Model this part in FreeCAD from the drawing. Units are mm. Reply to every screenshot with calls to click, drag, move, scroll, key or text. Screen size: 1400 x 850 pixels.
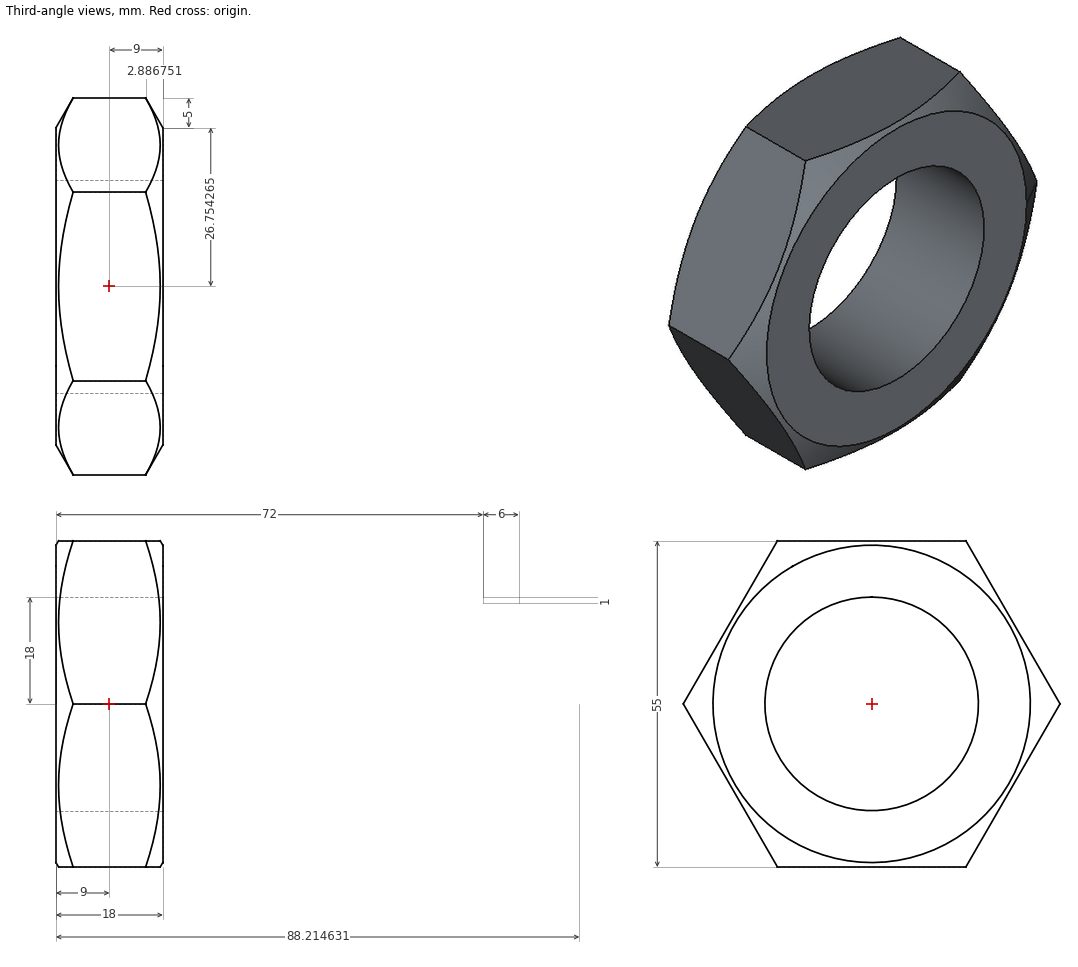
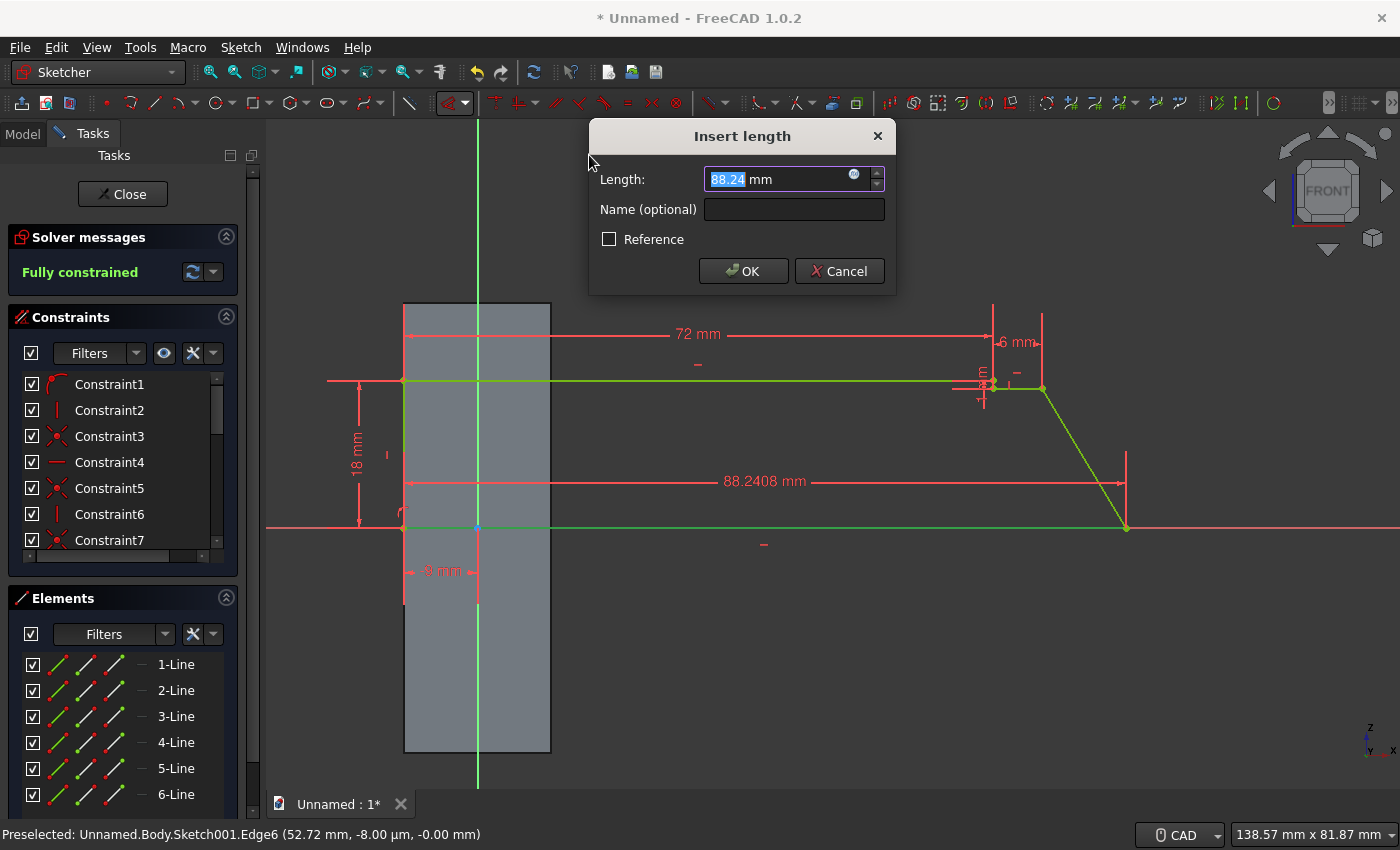
text(88.214631)
key(Return)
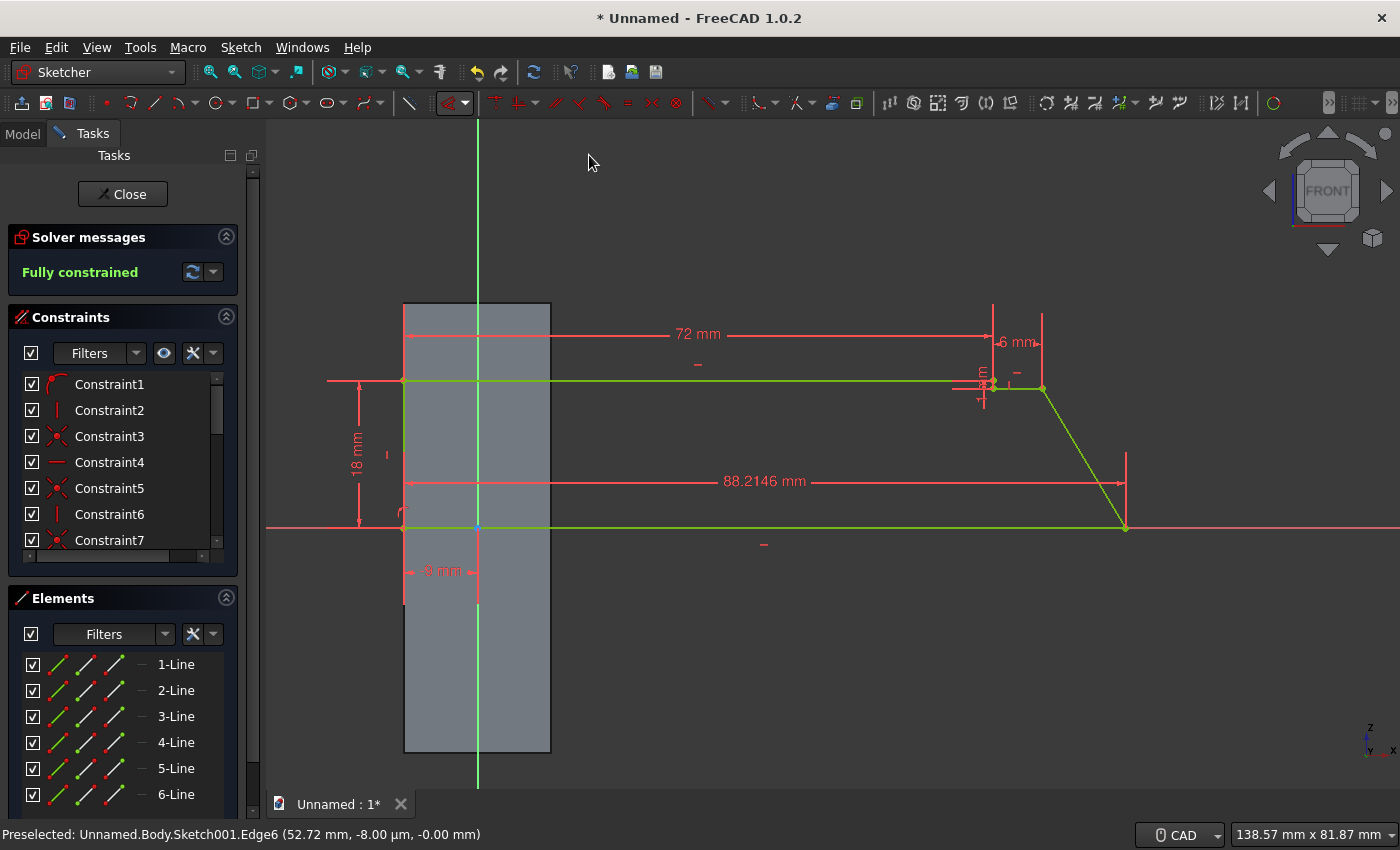
click(123, 194)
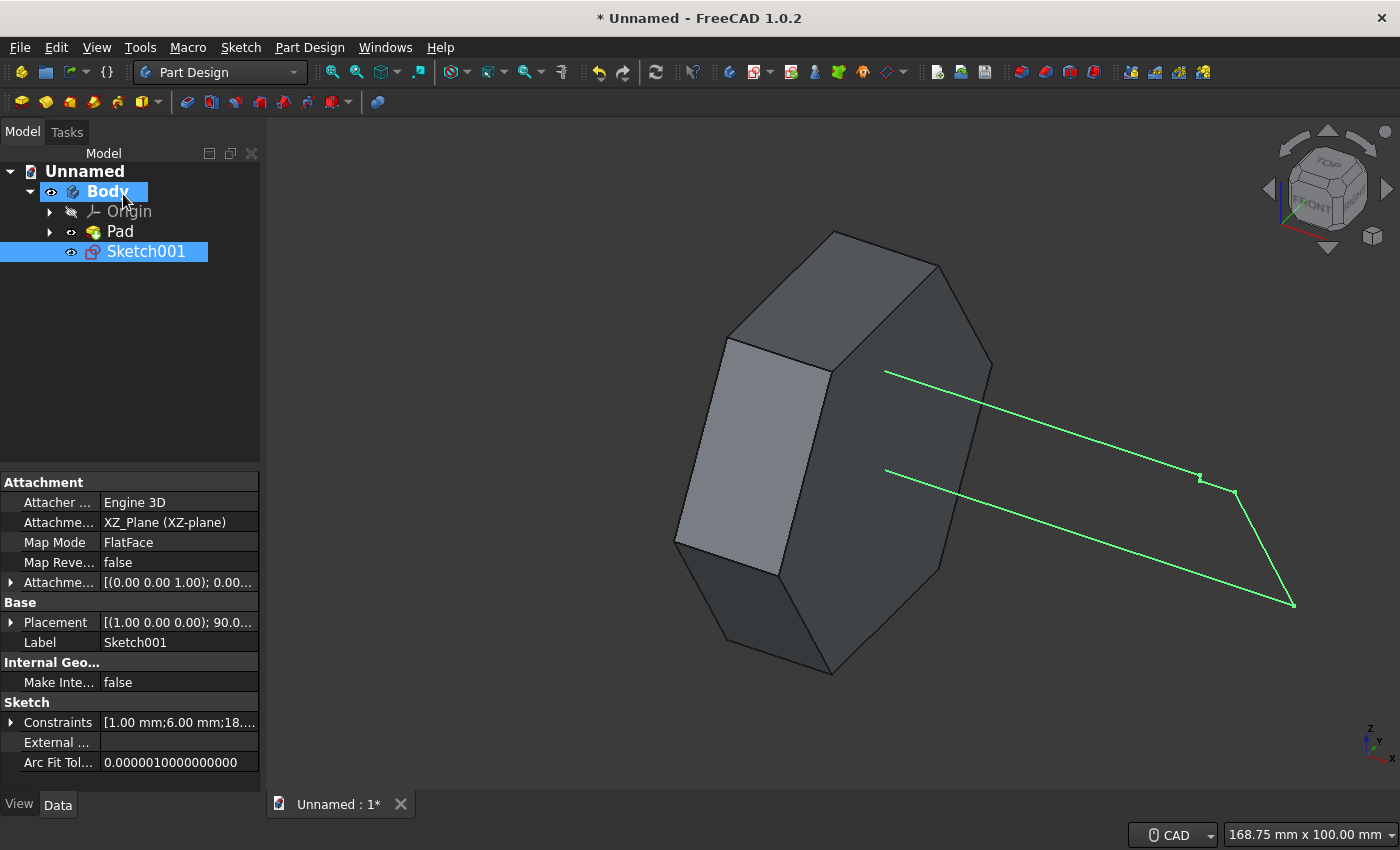
click(236, 102)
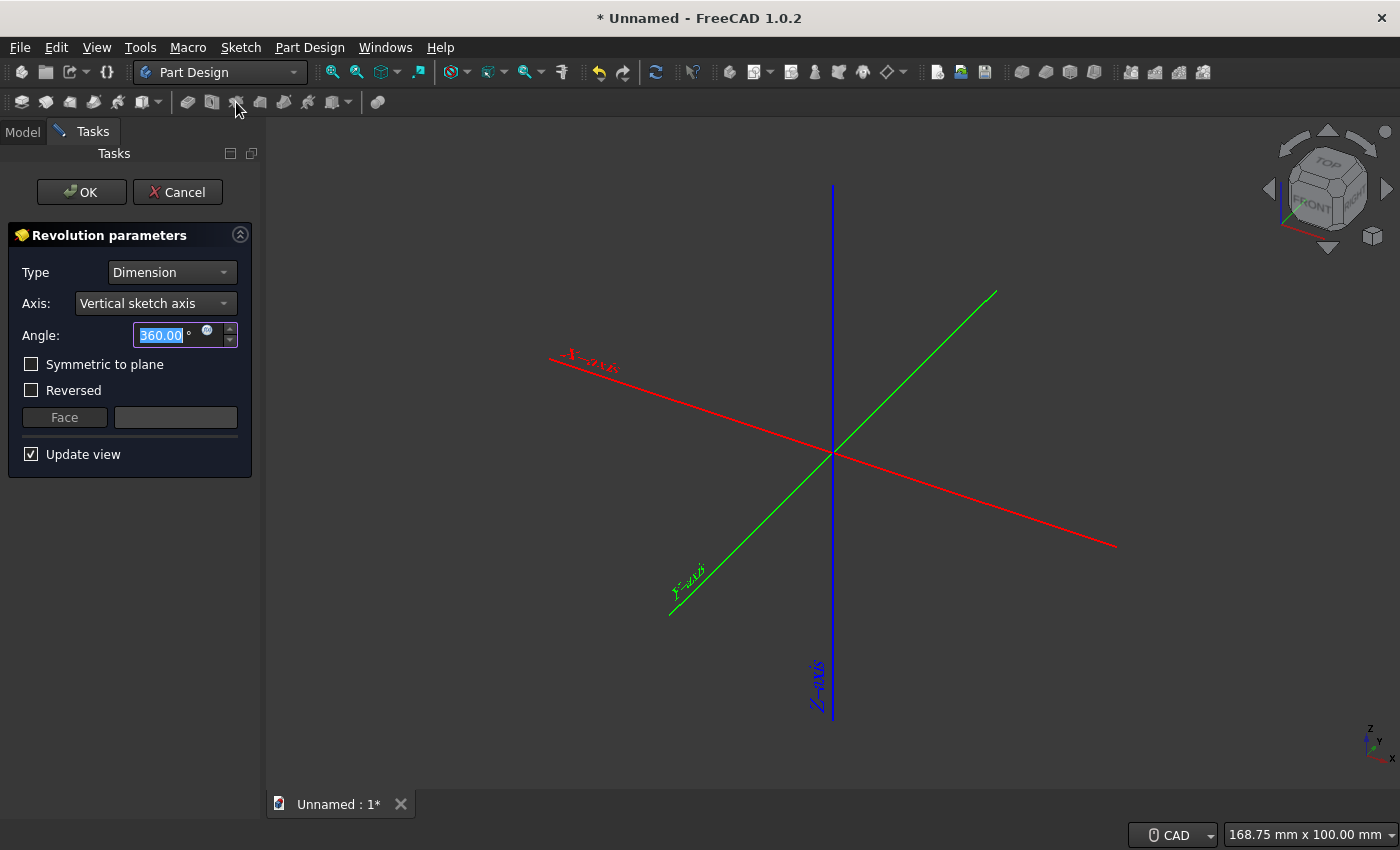
click(156, 304)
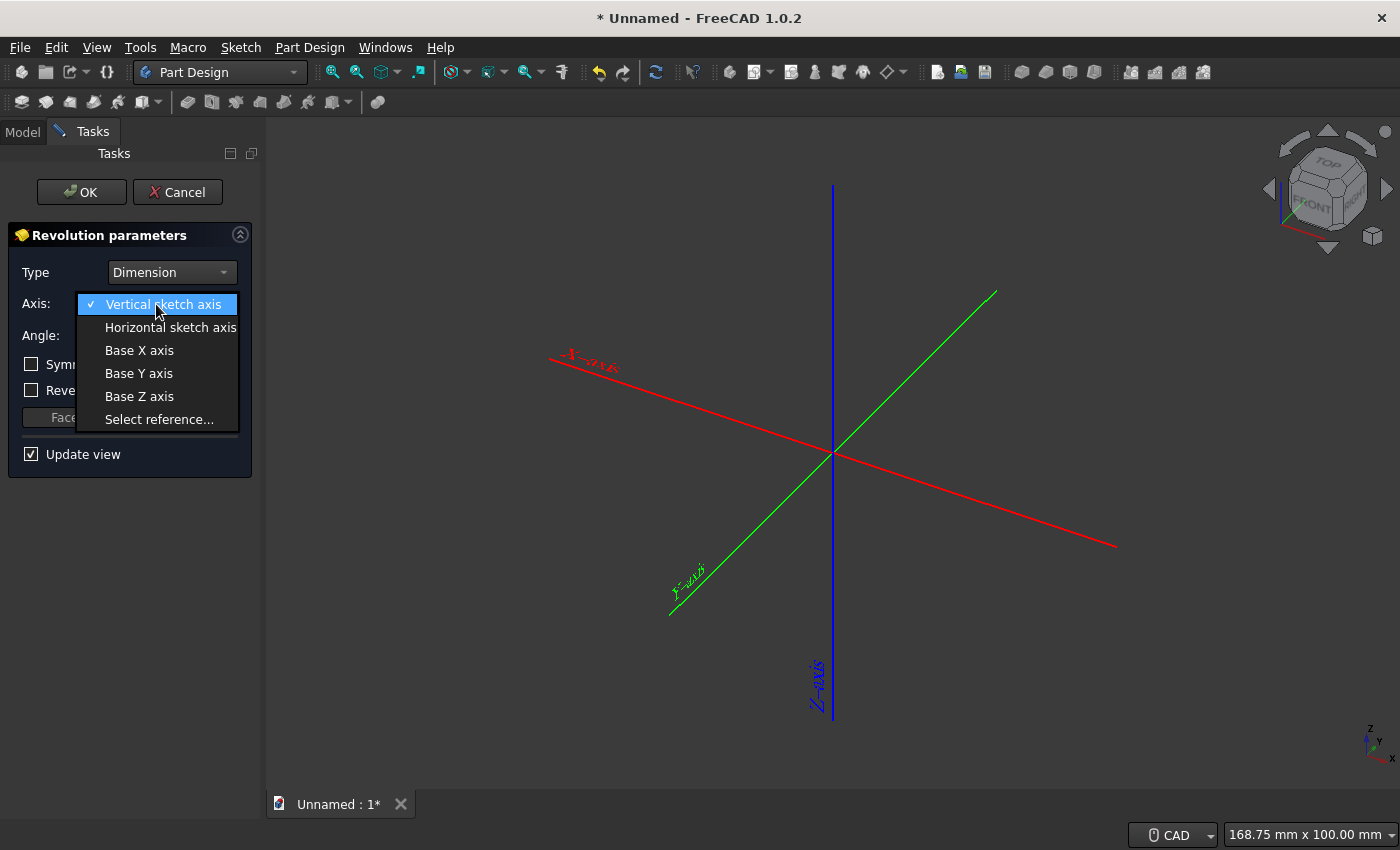
click(156, 328)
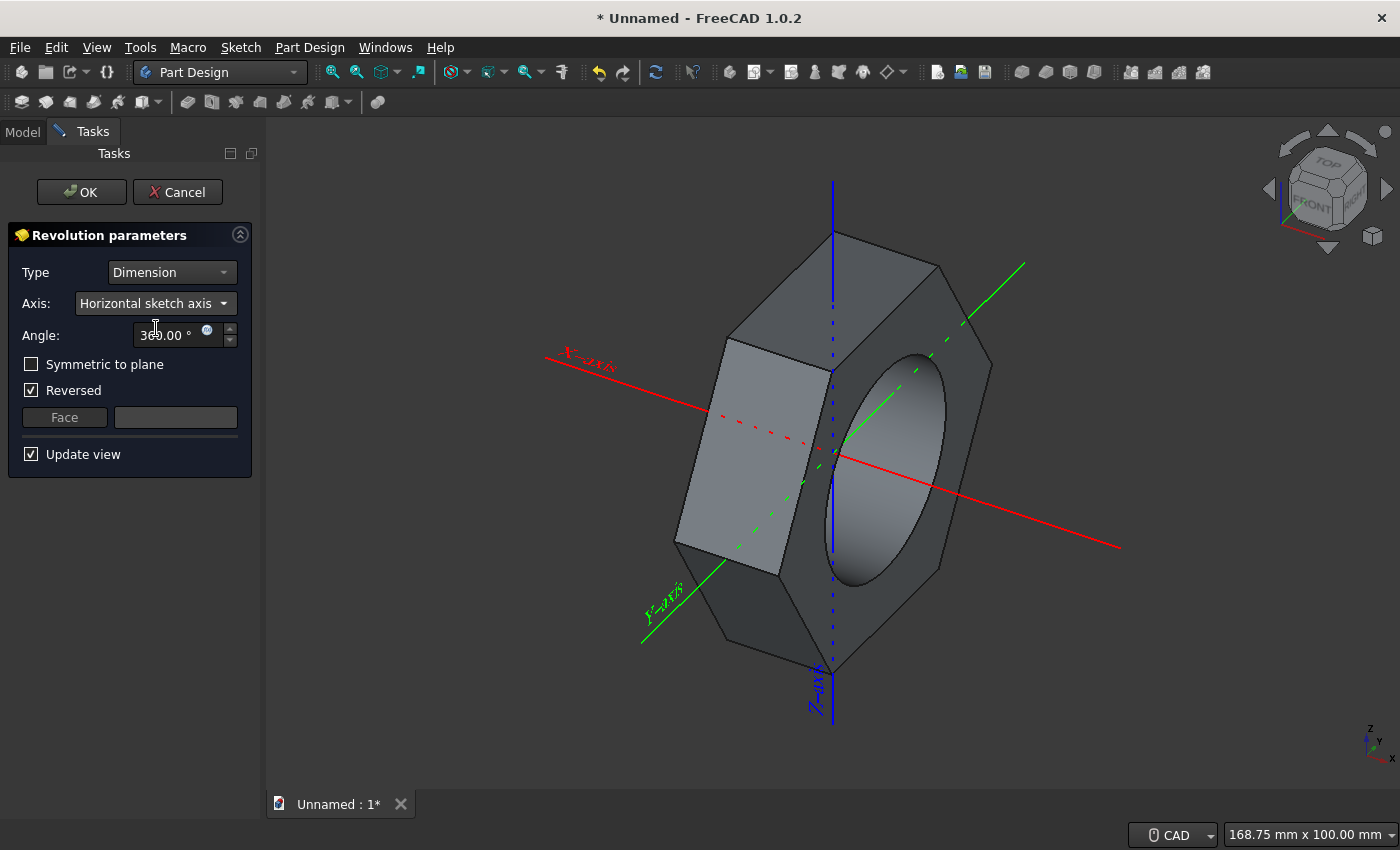
click(82, 192)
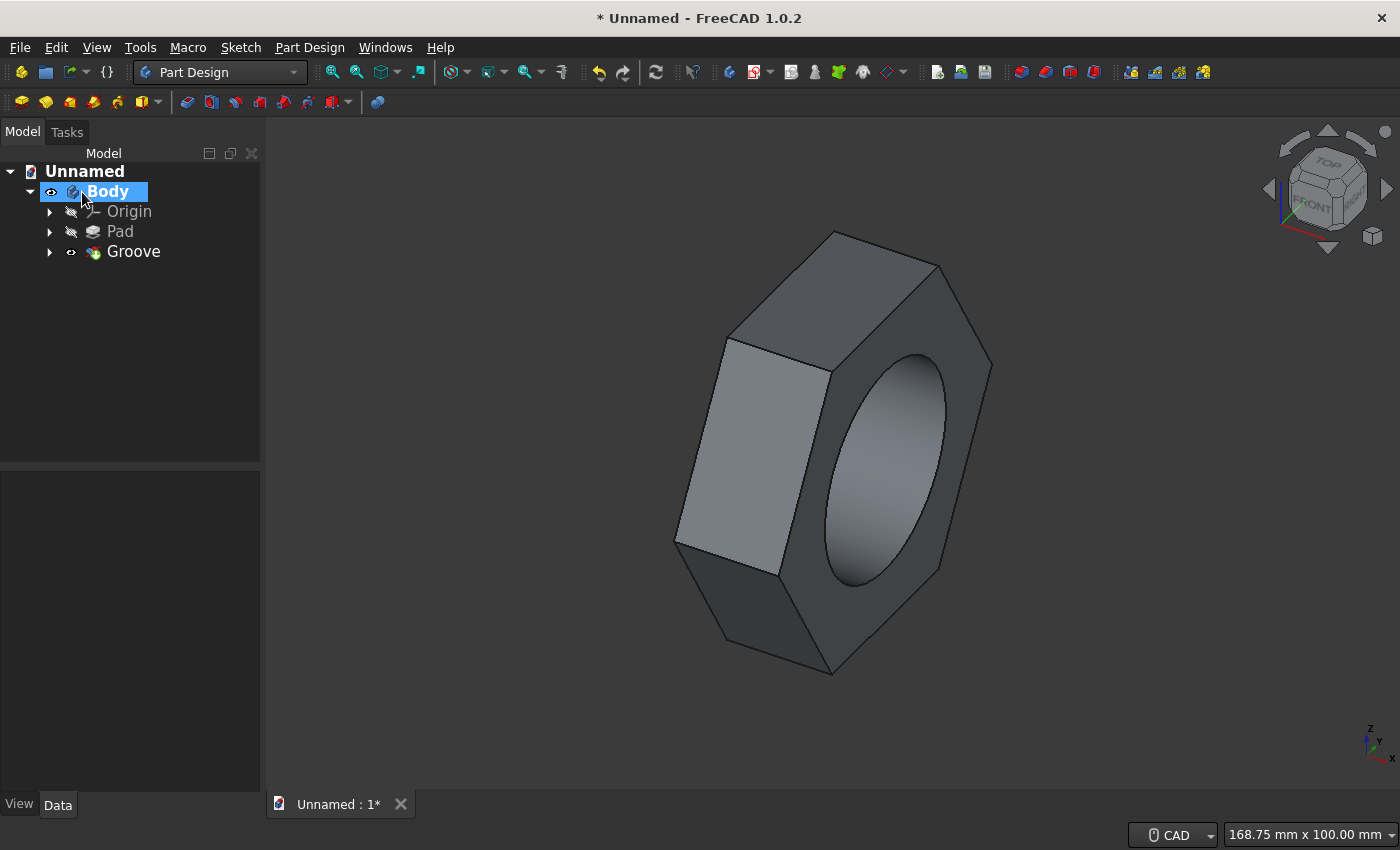
click(754, 72)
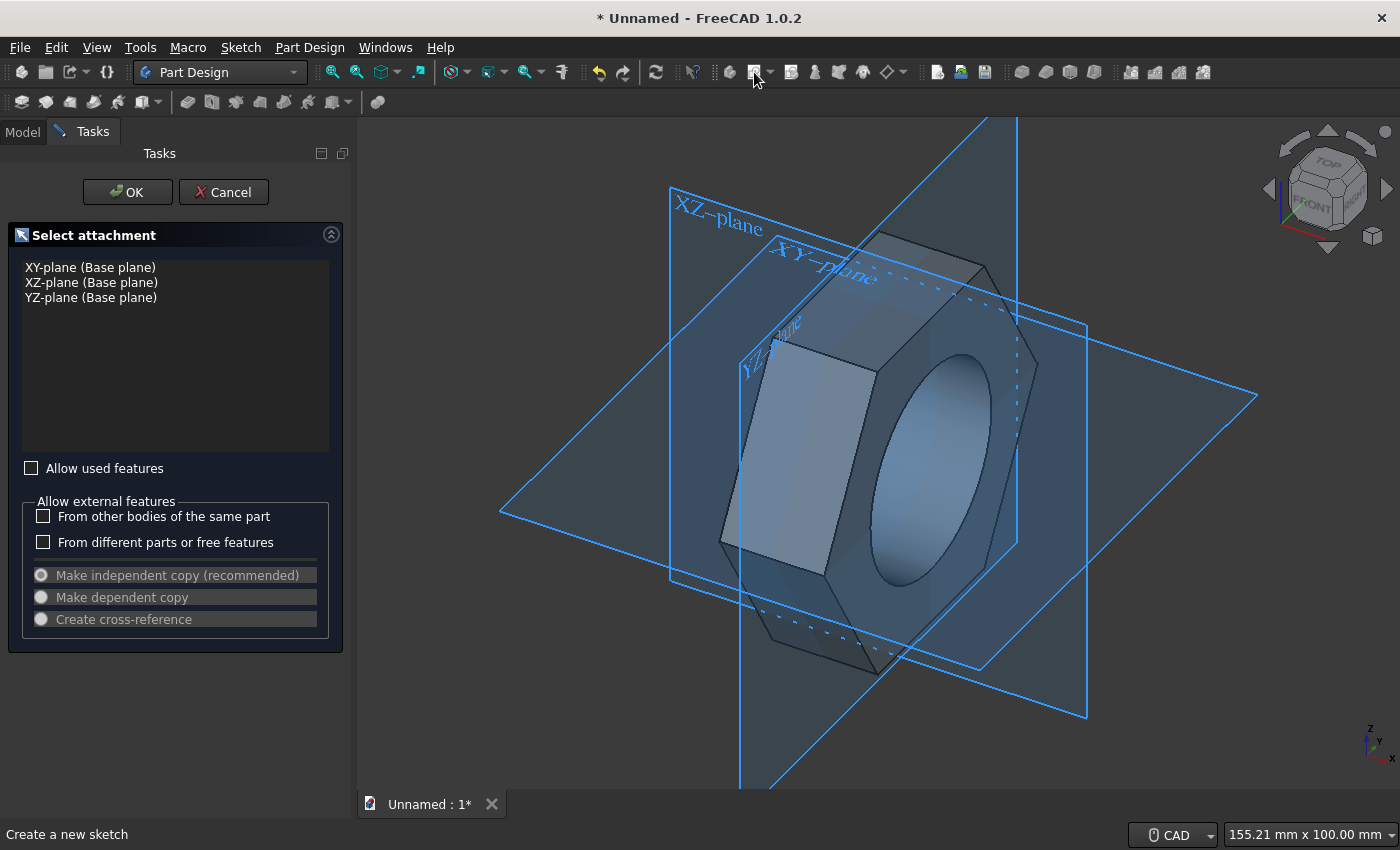
click(82, 268)